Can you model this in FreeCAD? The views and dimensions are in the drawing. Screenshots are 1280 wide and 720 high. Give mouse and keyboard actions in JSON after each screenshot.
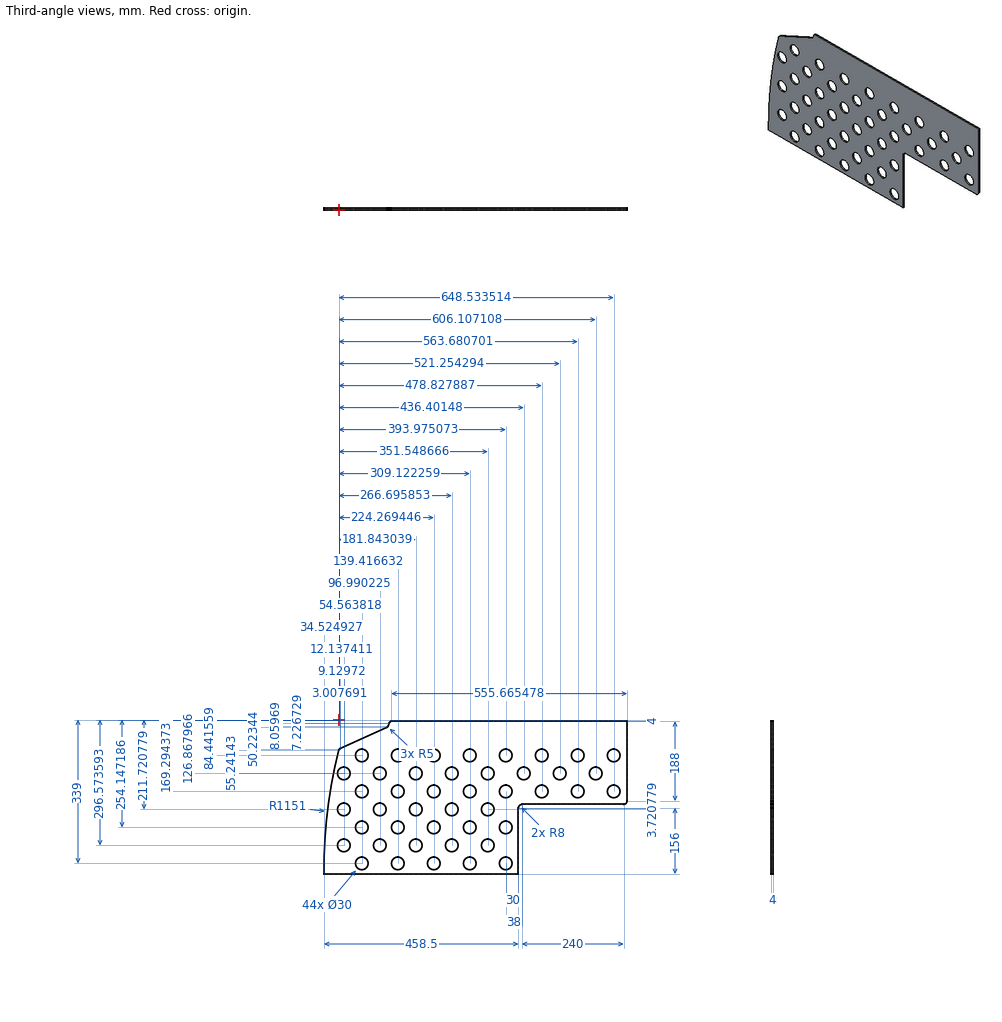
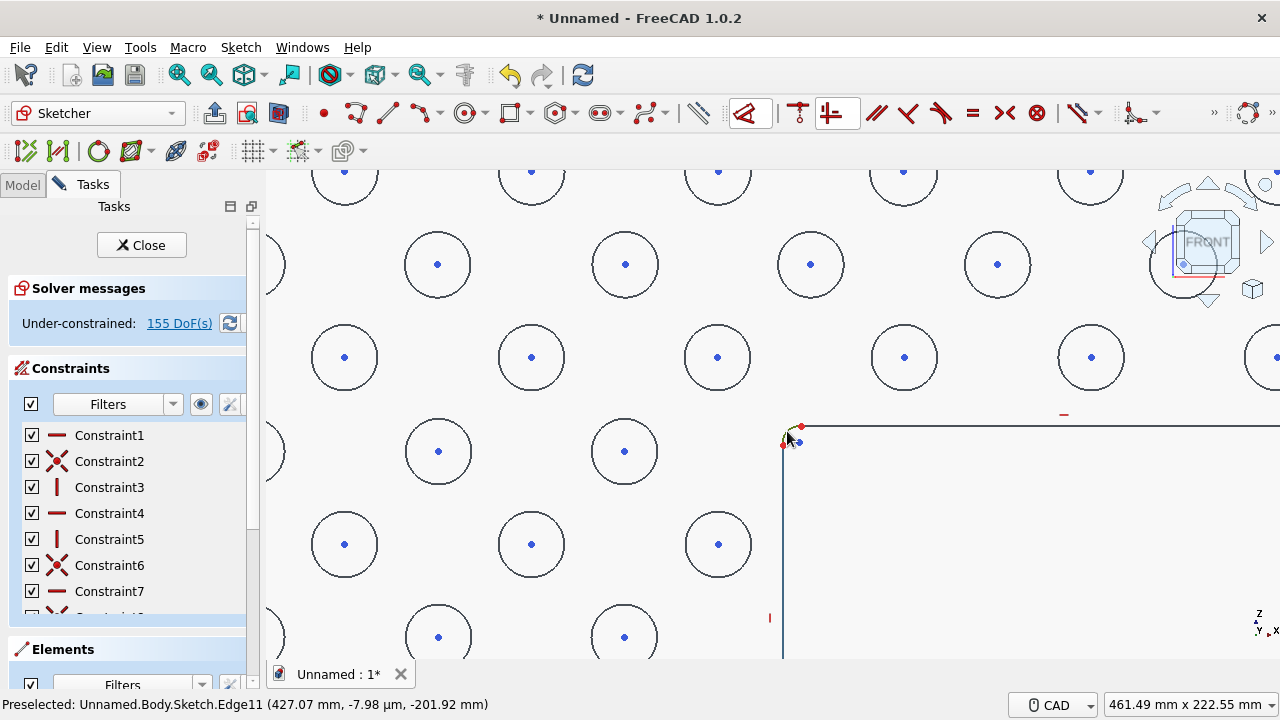
{"action": "left_click", "coordinate": [942, 114]}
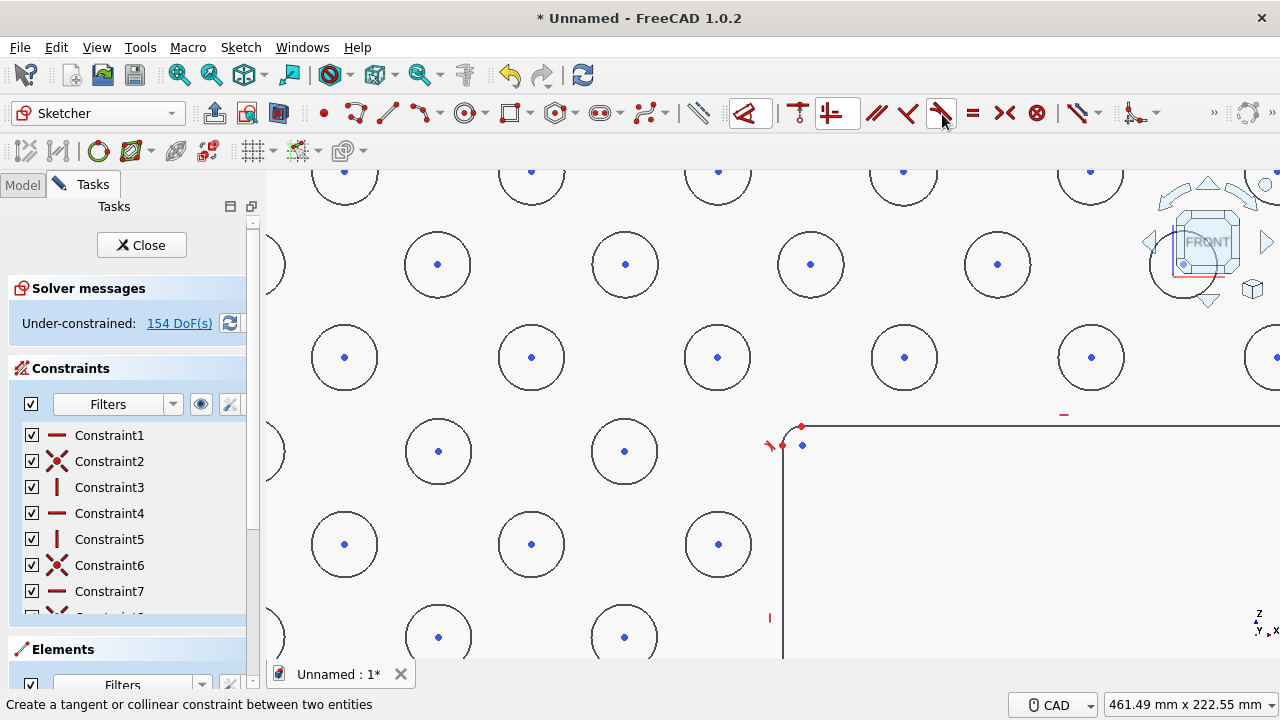
{"action": "left_click", "coordinate": [959, 426]}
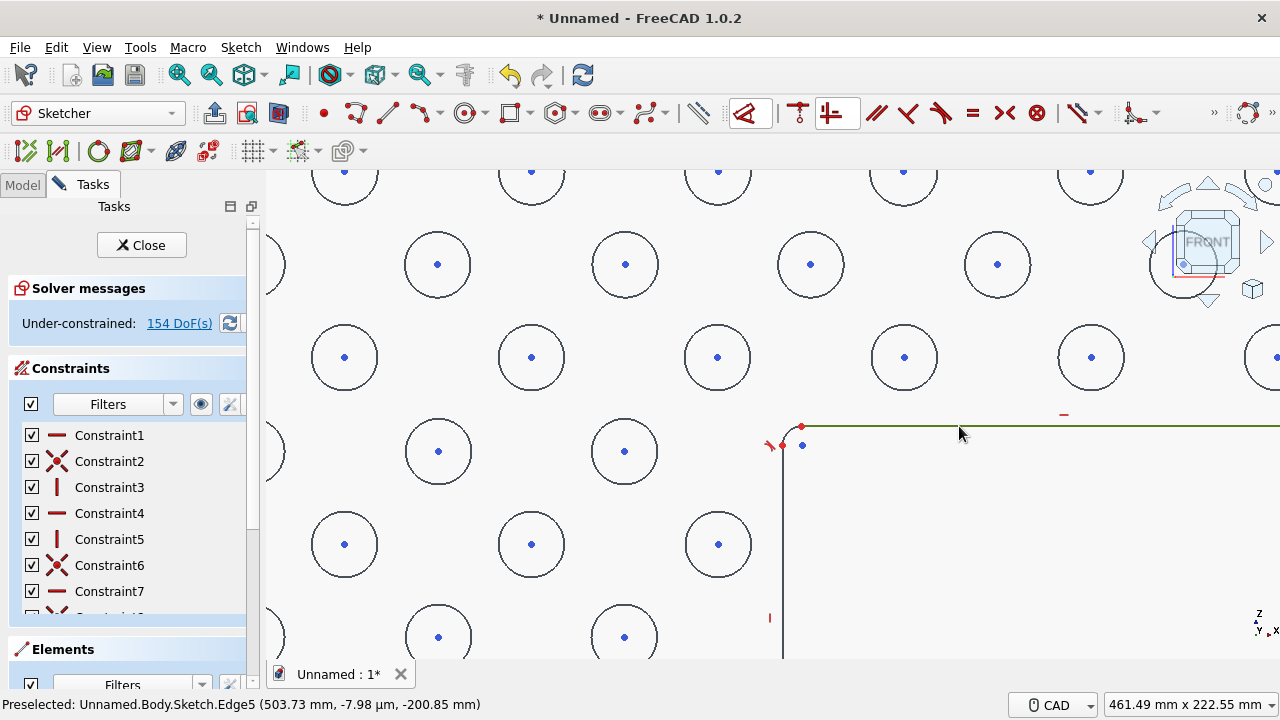
{"action": "left_click", "coordinate": [788, 432]}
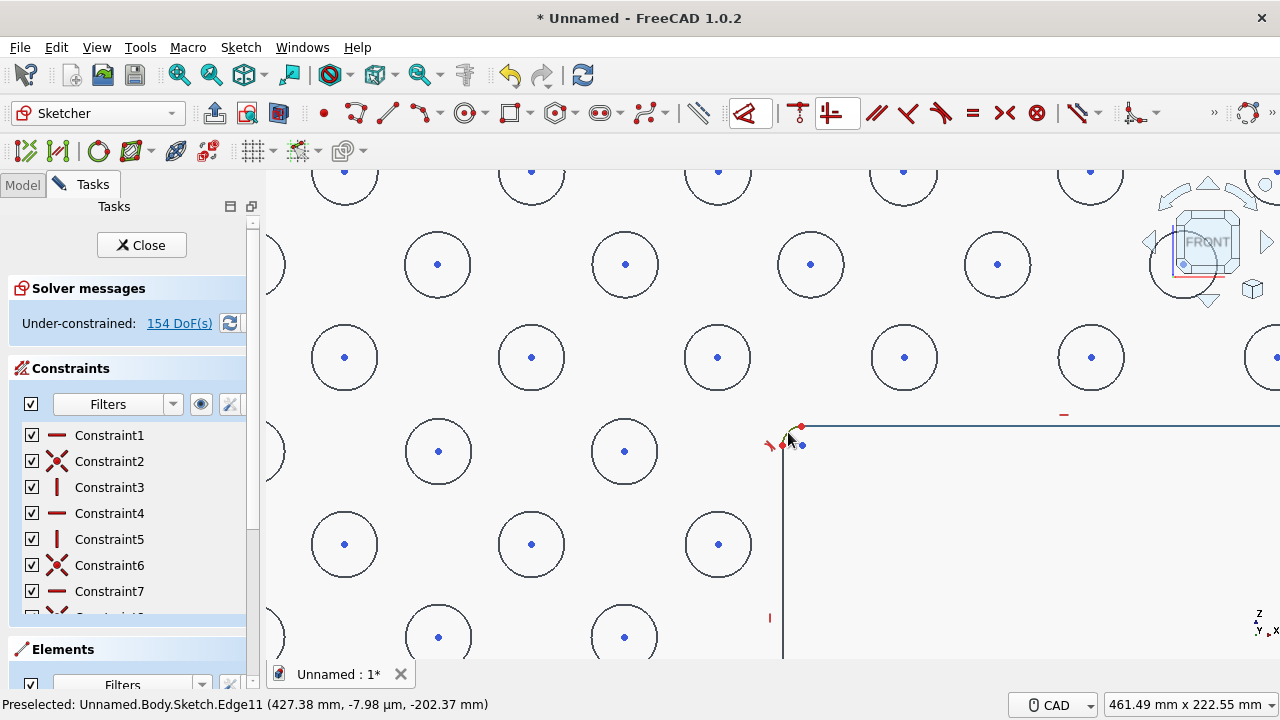
{"action": "key", "text": "t"}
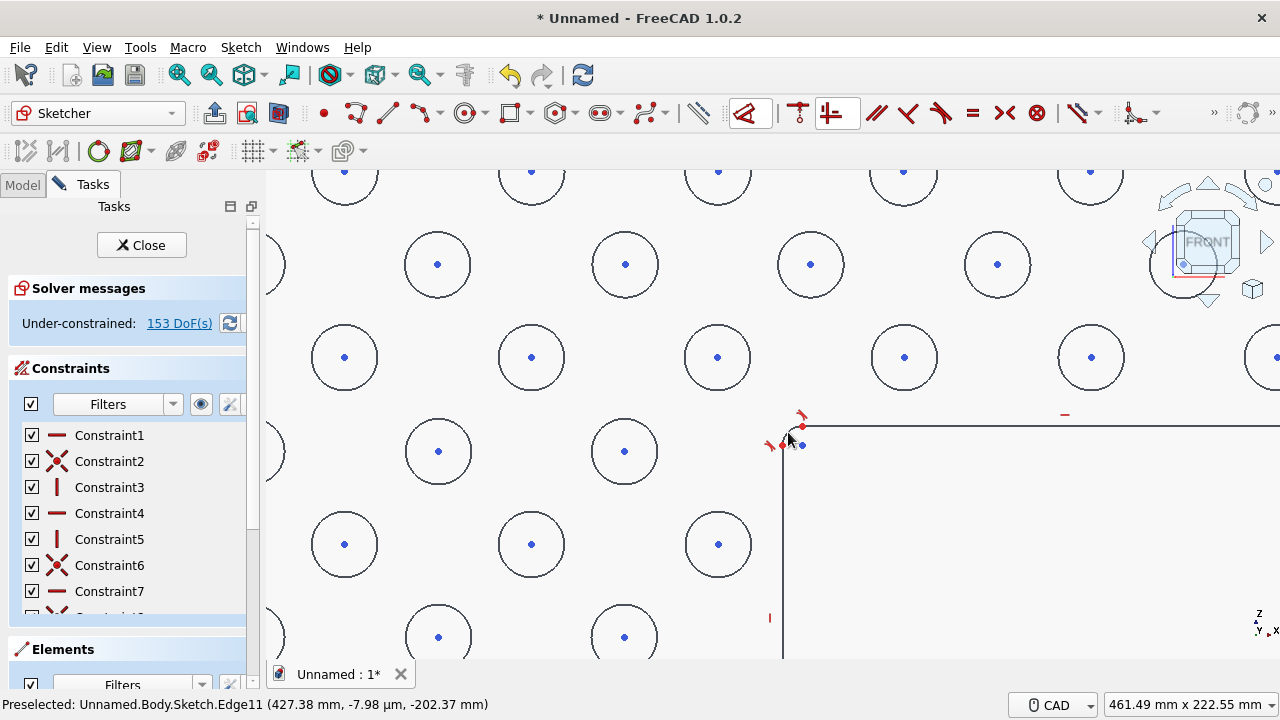
{"action": "left_click", "coordinate": [960, 426]}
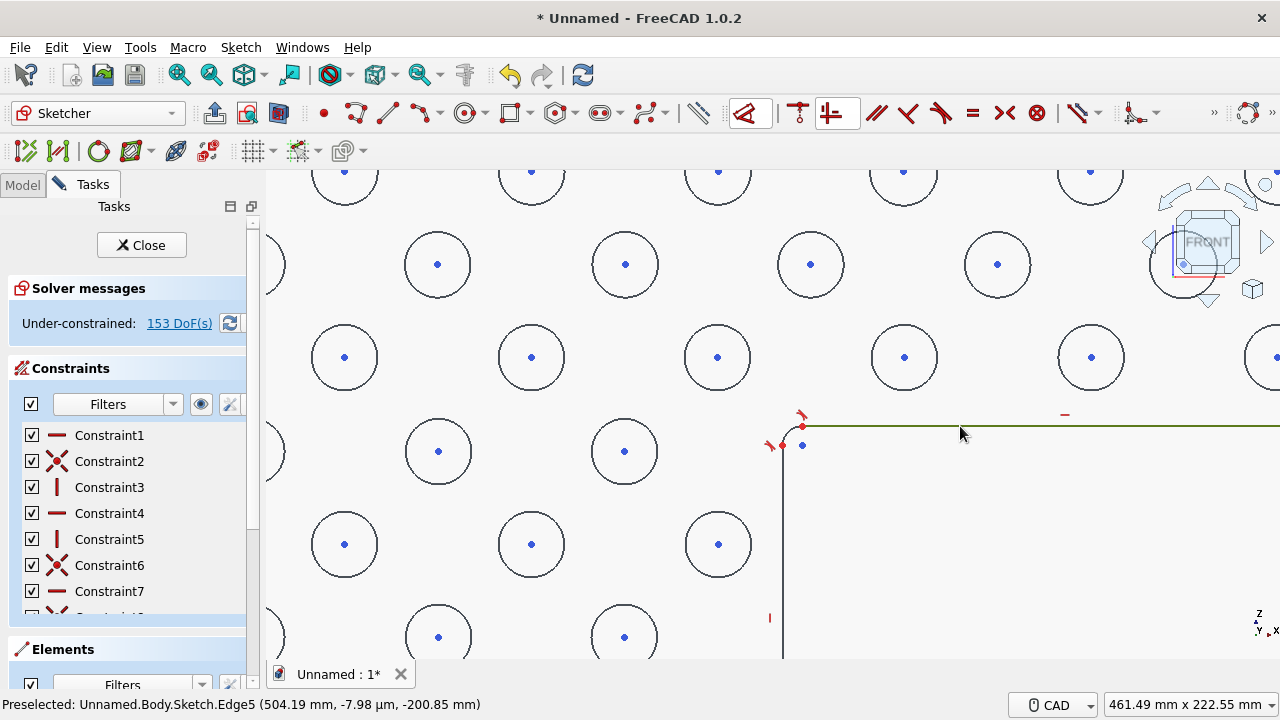
{"action": "scroll", "coordinate": [788, 432], "scroll_direction": "down", "scroll_amount": 5}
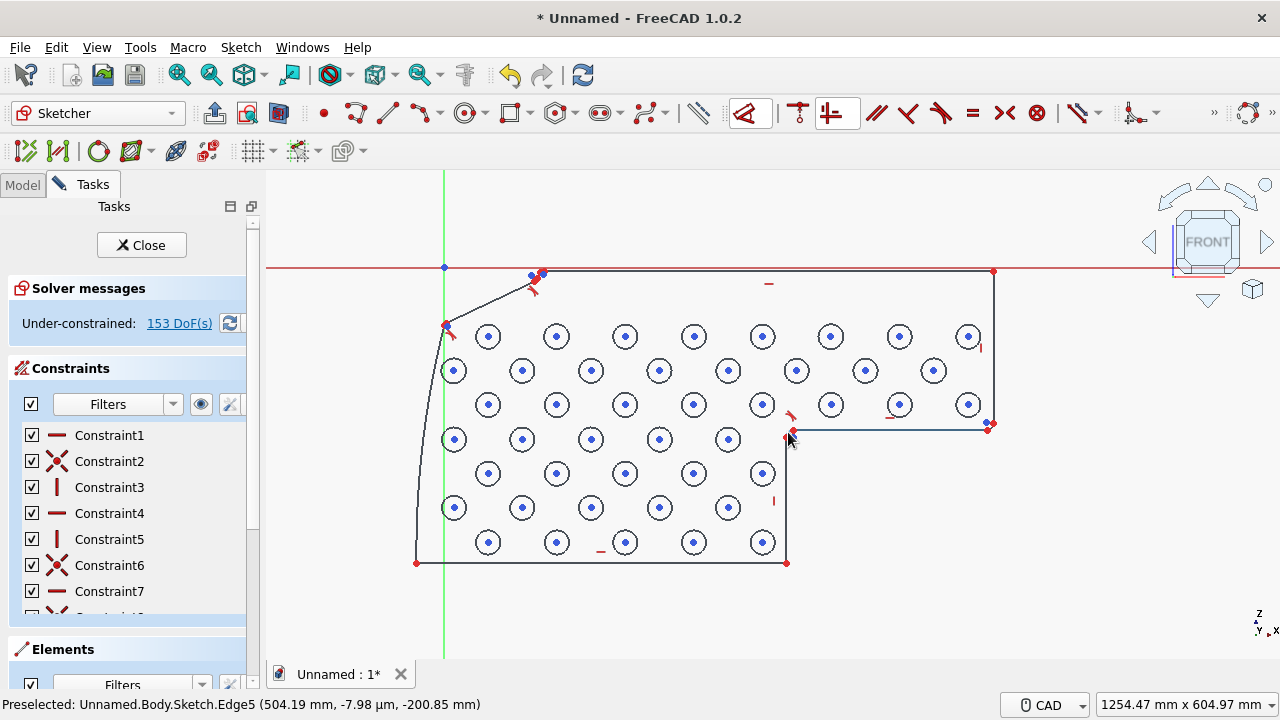
{"action": "scroll", "coordinate": [992, 428], "scroll_direction": "up", "scroll_amount": 6}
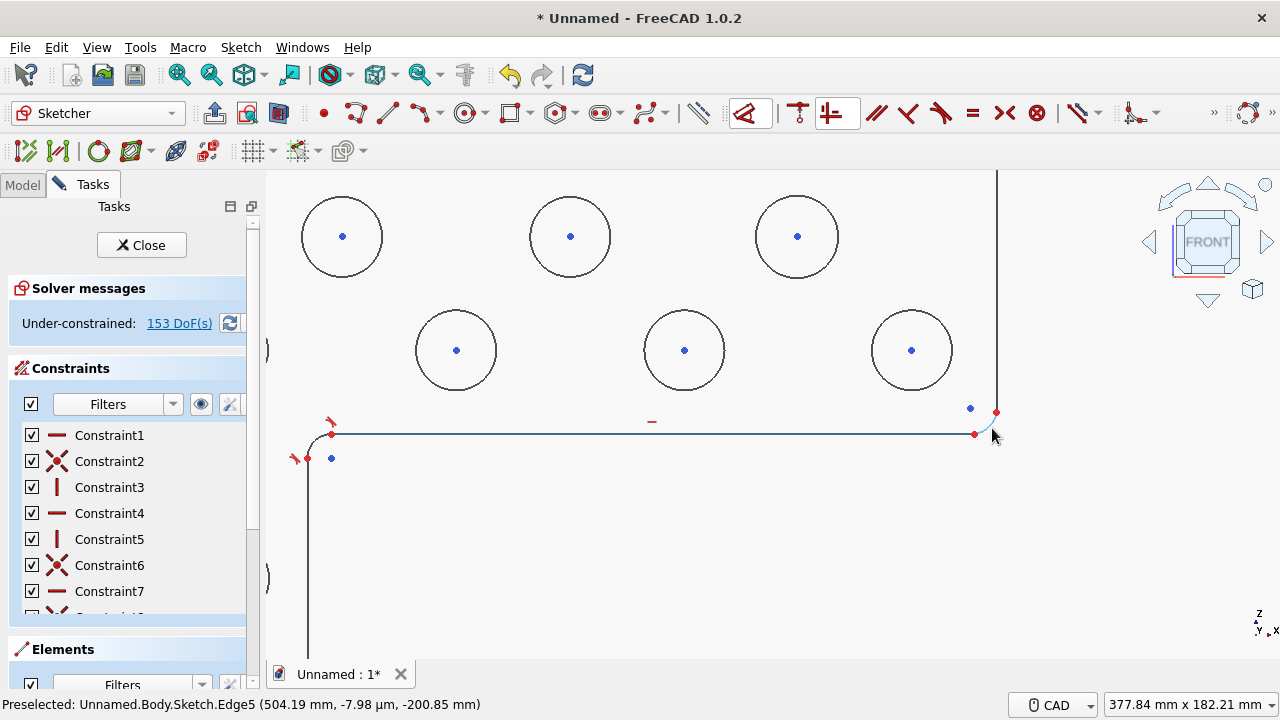
{"action": "left_click", "coordinate": [989, 427]}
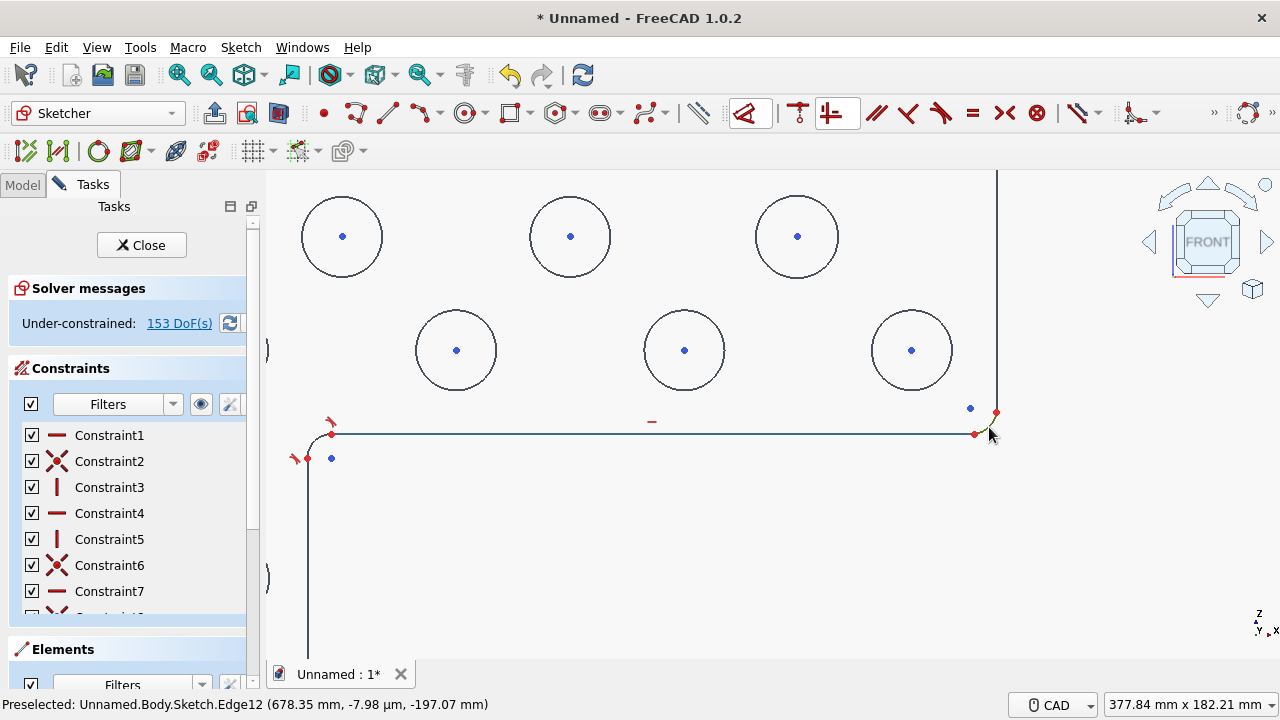
{"action": "left_click", "coordinate": [942, 114]}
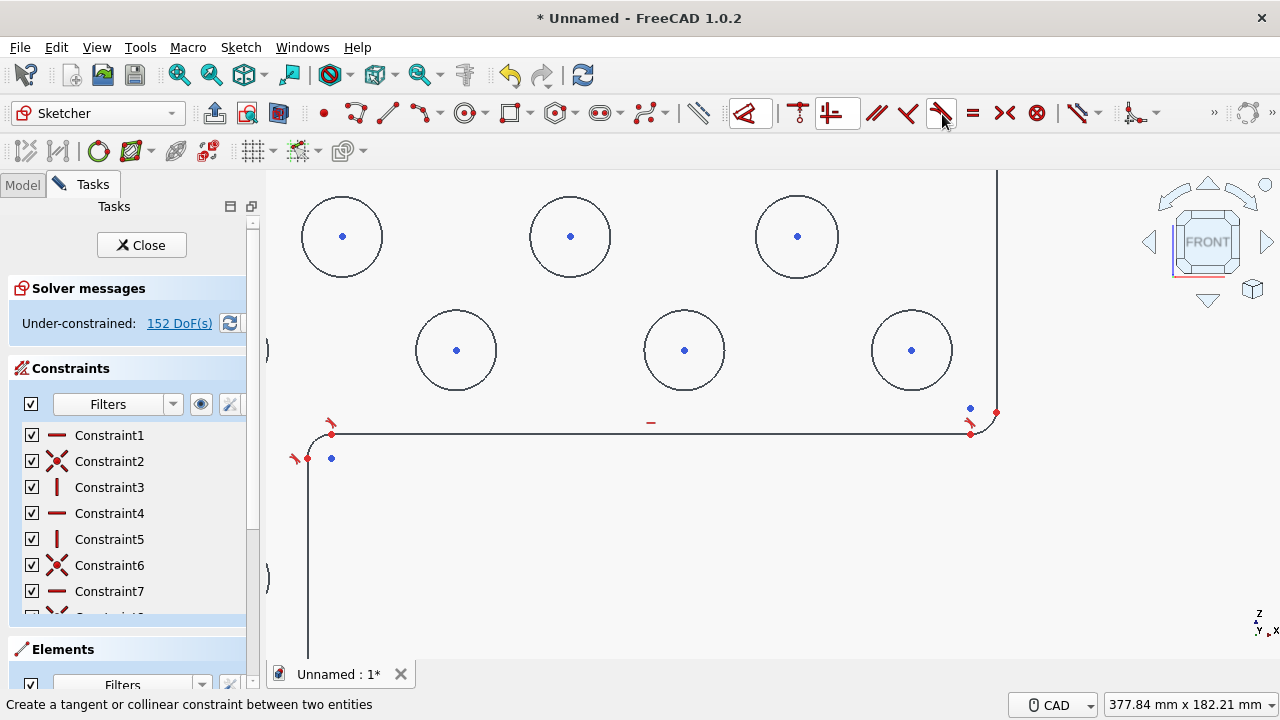
{"action": "left_click", "coordinate": [997, 261]}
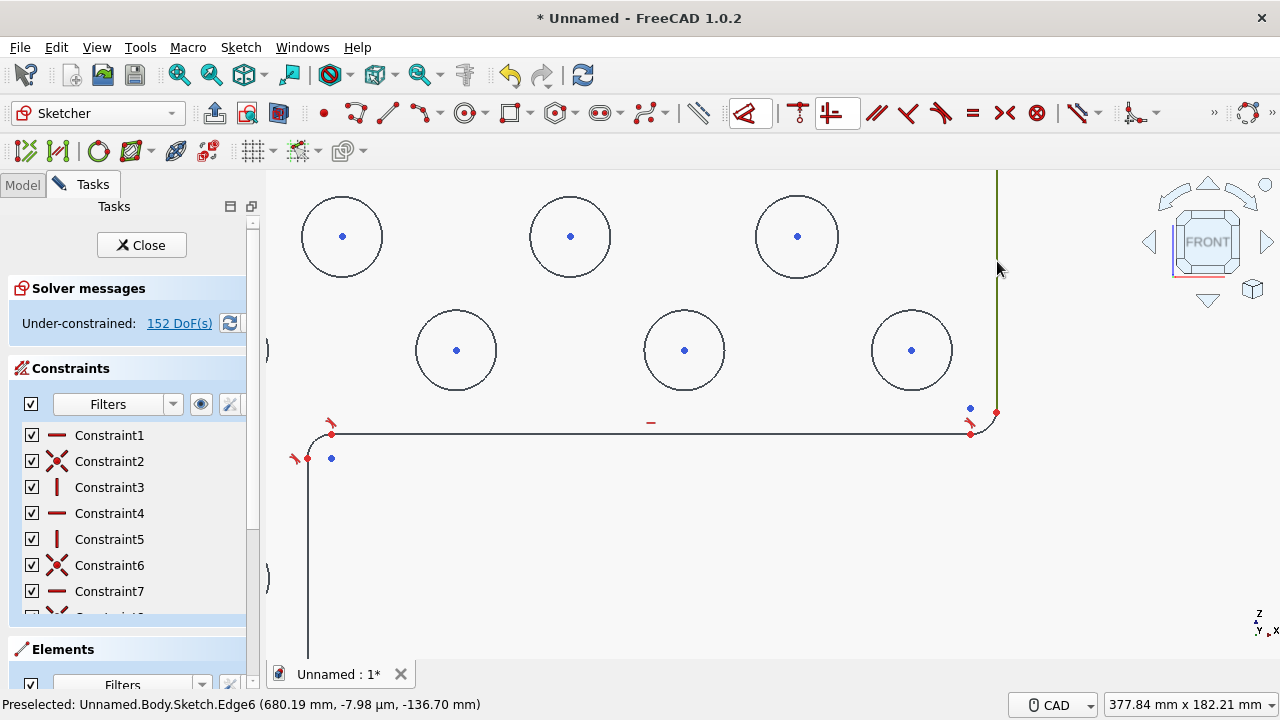
{"action": "scroll", "coordinate": [982, 432], "scroll_direction": "up", "scroll_amount": 2}